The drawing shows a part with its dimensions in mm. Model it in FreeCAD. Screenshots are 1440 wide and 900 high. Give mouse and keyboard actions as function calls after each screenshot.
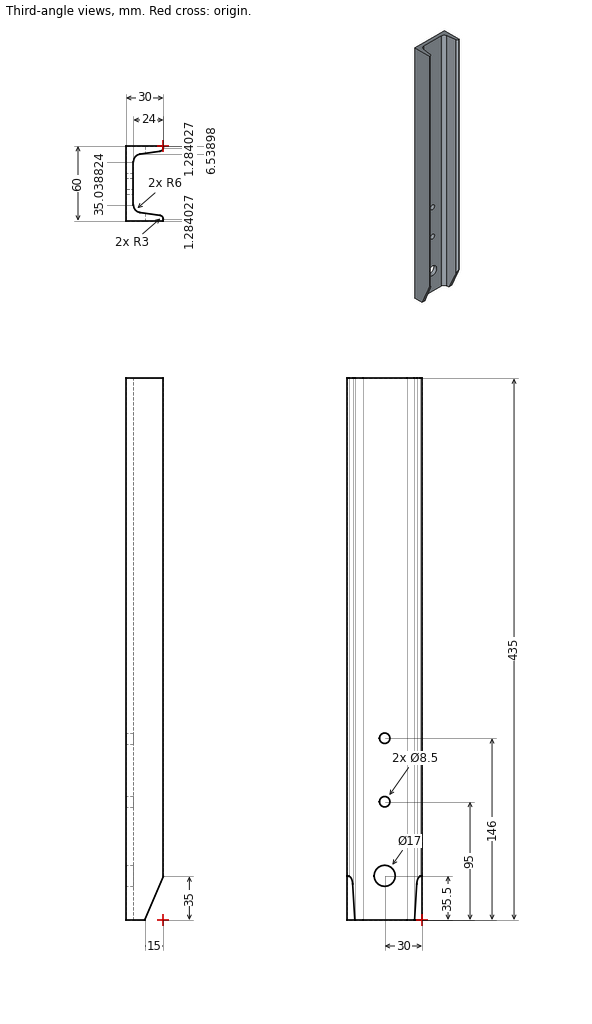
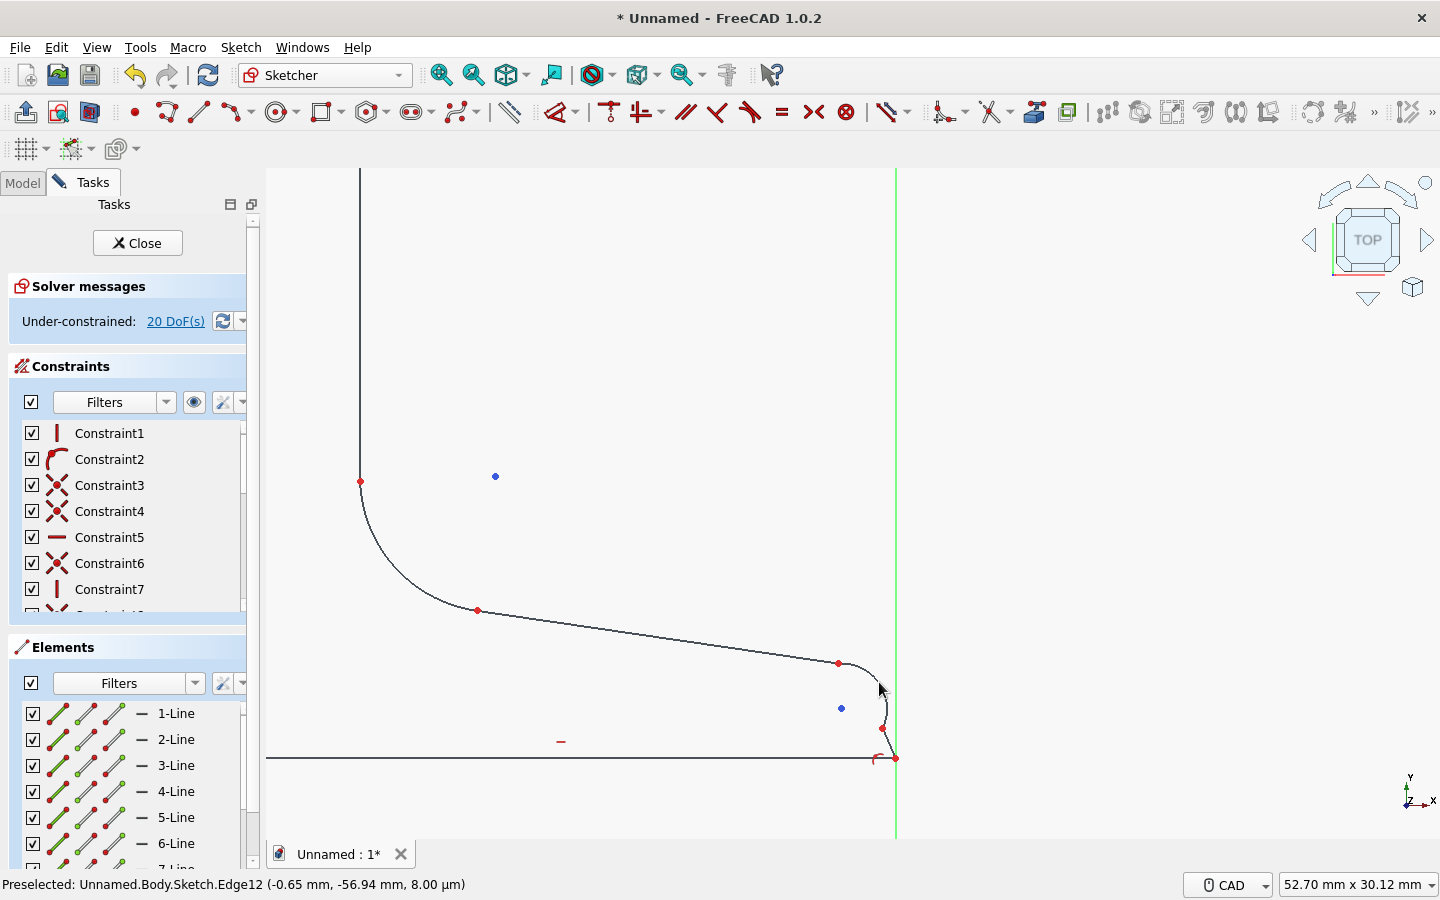
scroll(881, 683, down, 6)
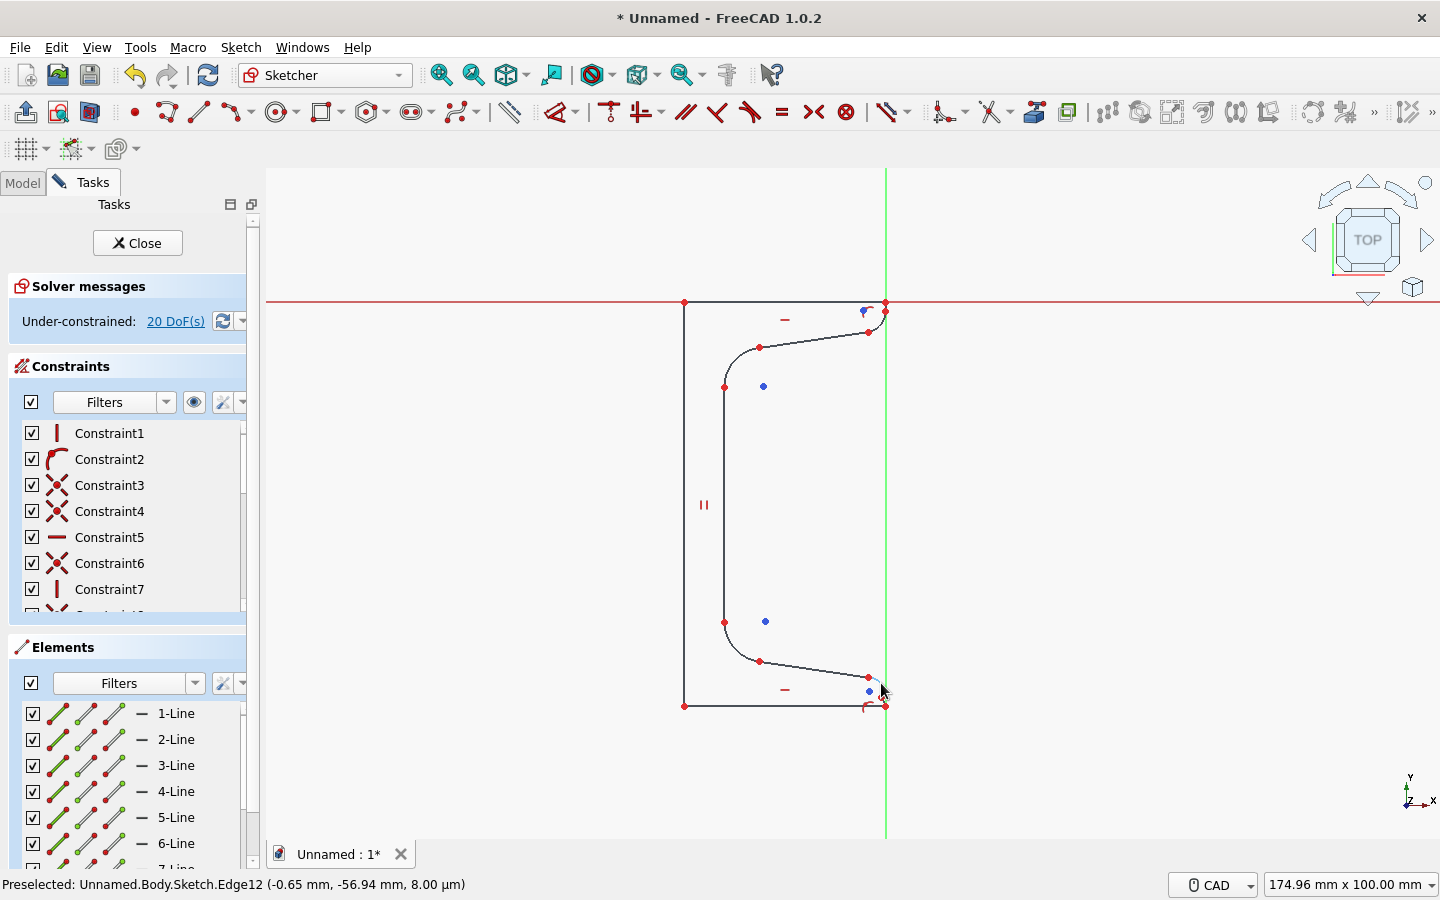
click(836, 673)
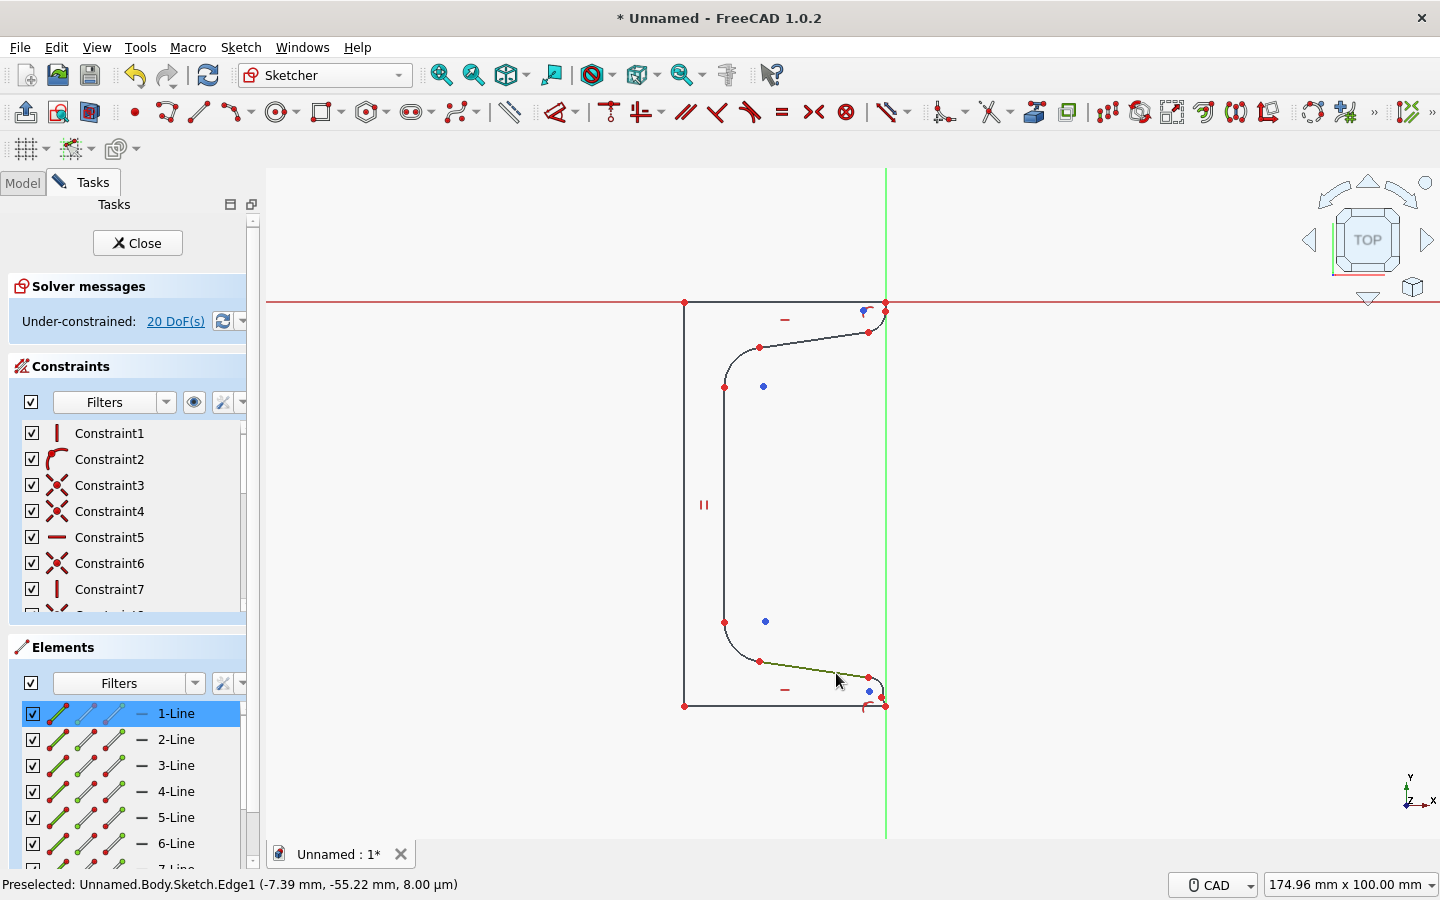
click(729, 639)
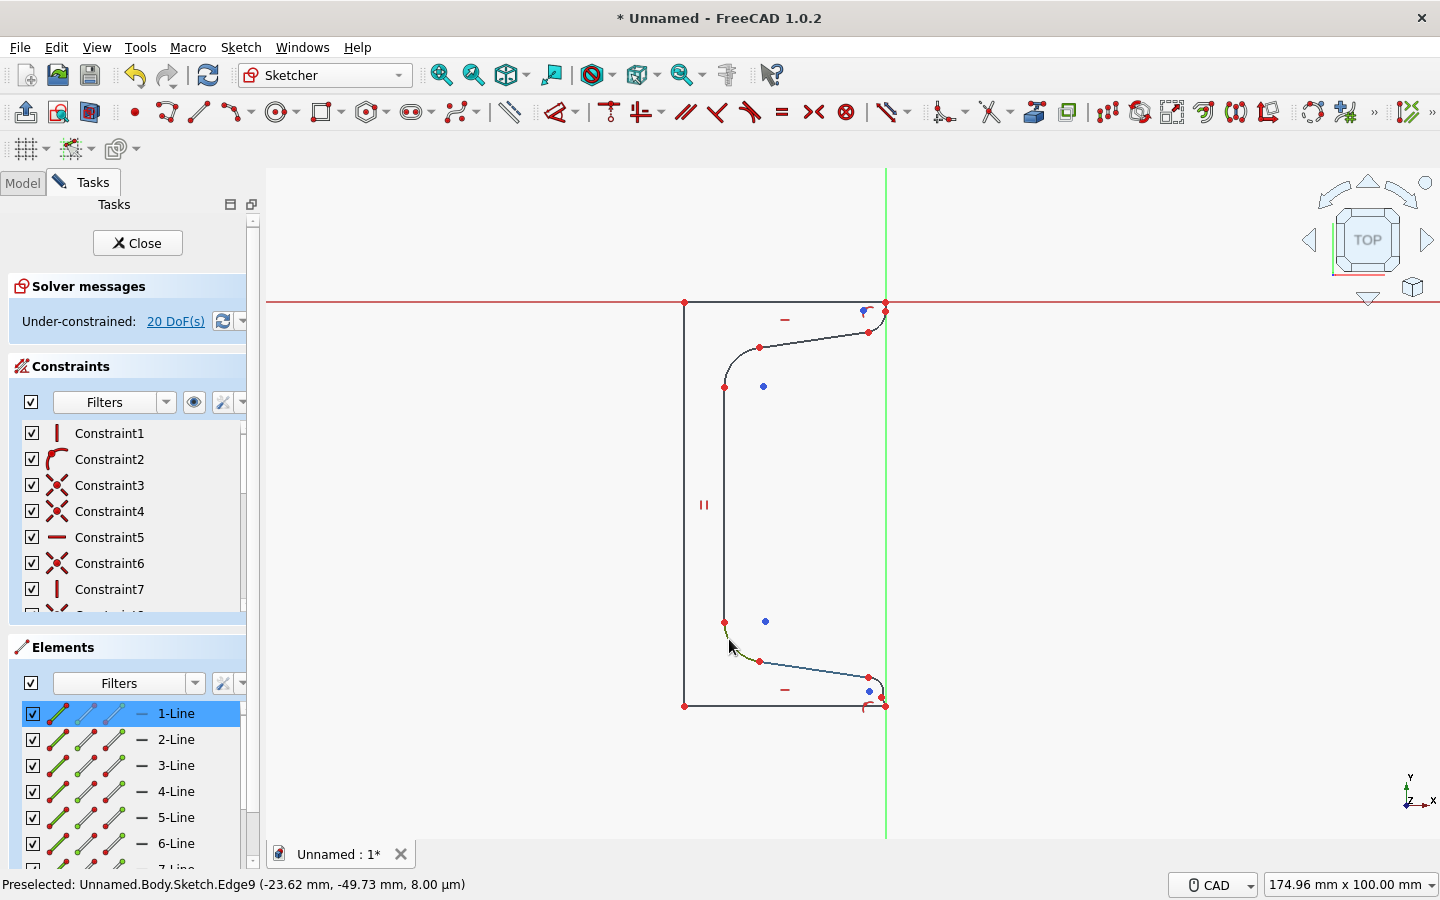
click(750, 112)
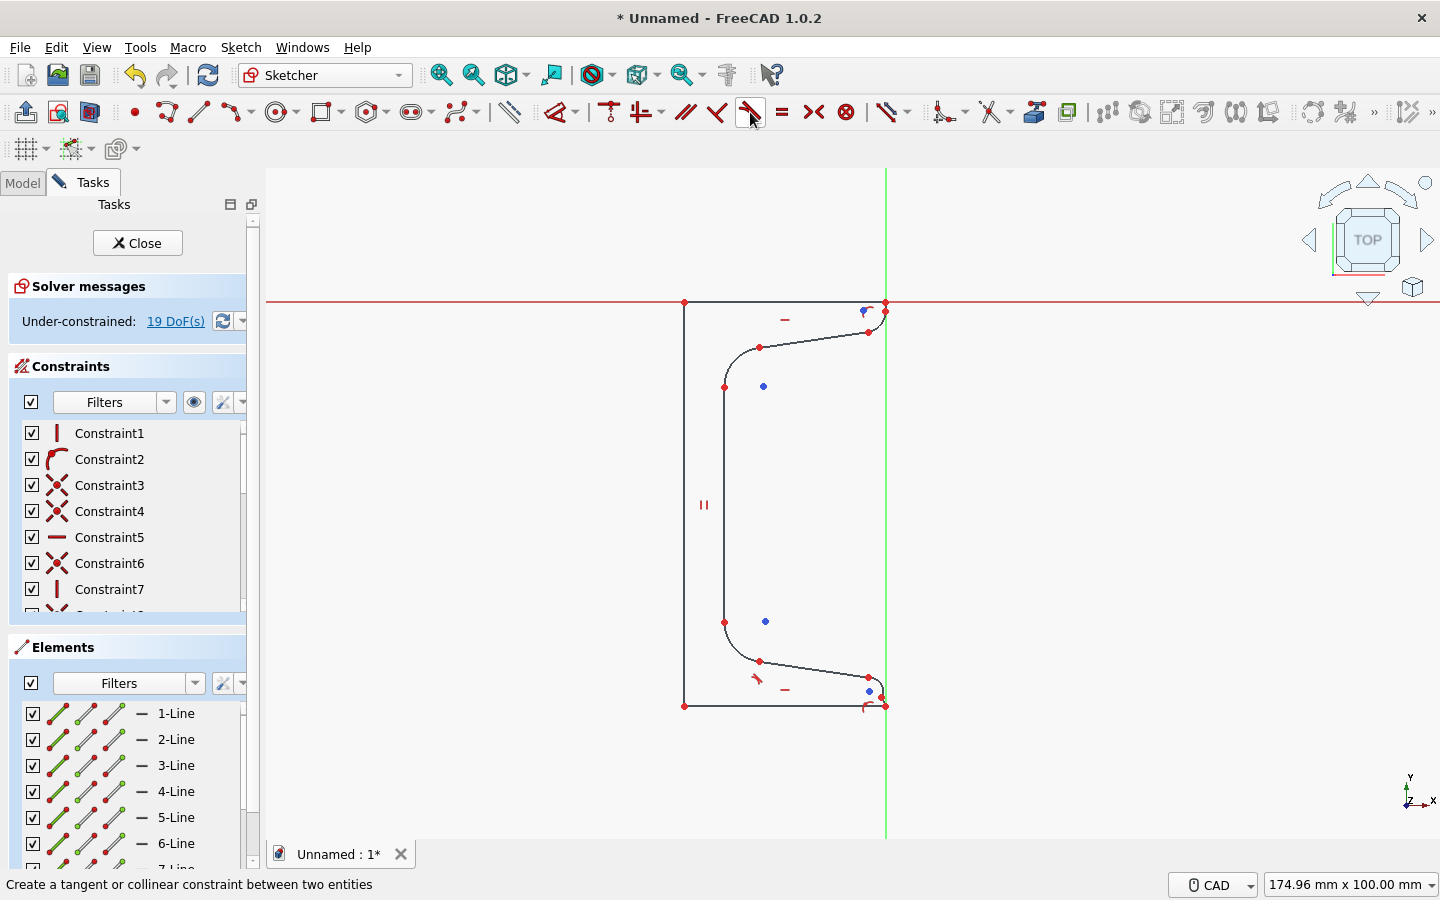
click(836, 673)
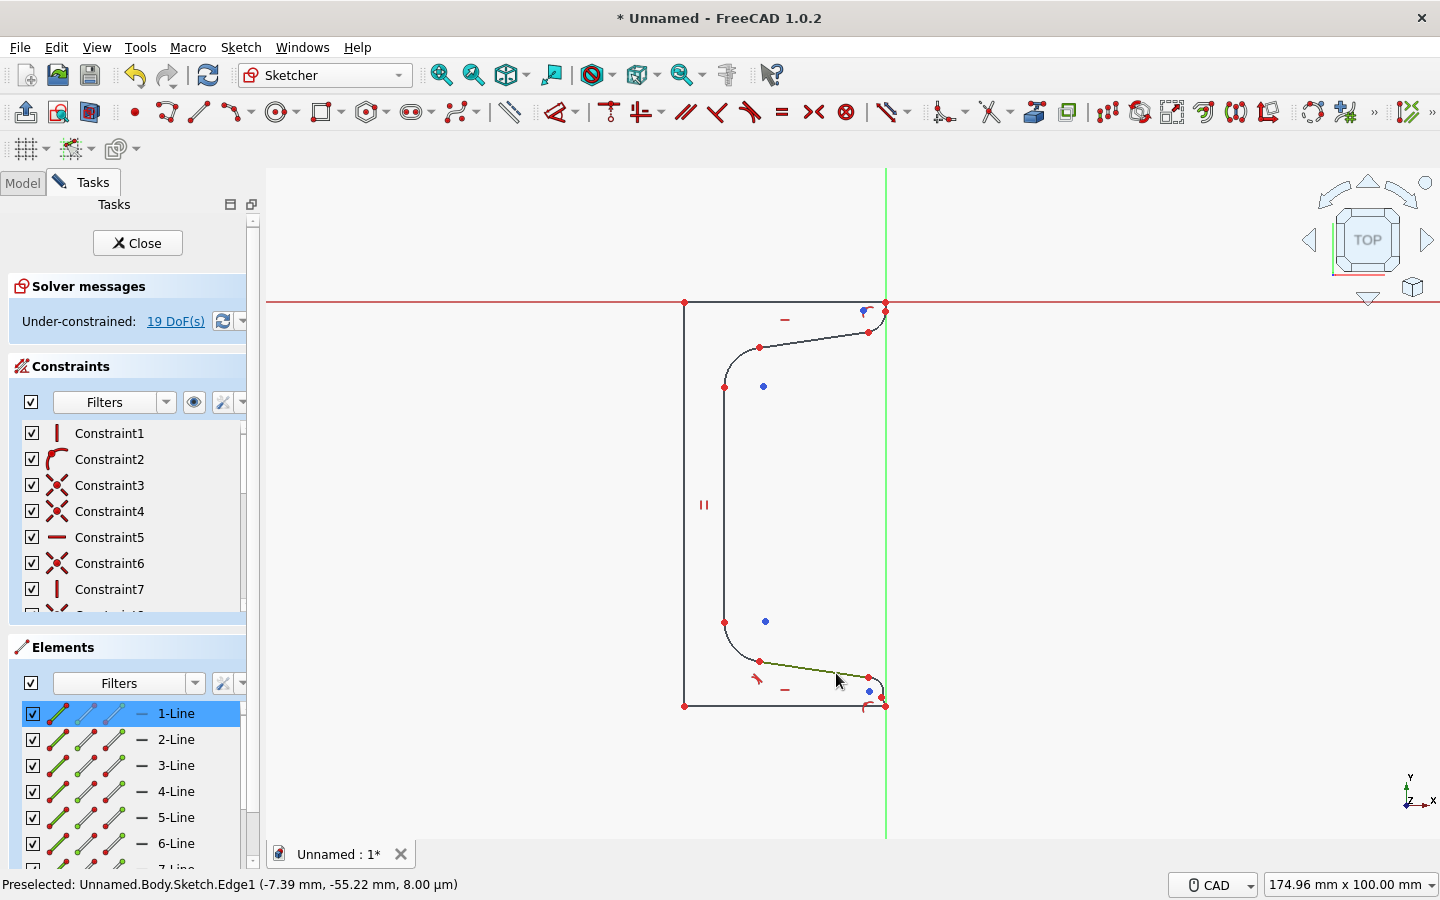
scroll(877, 680, up, 3)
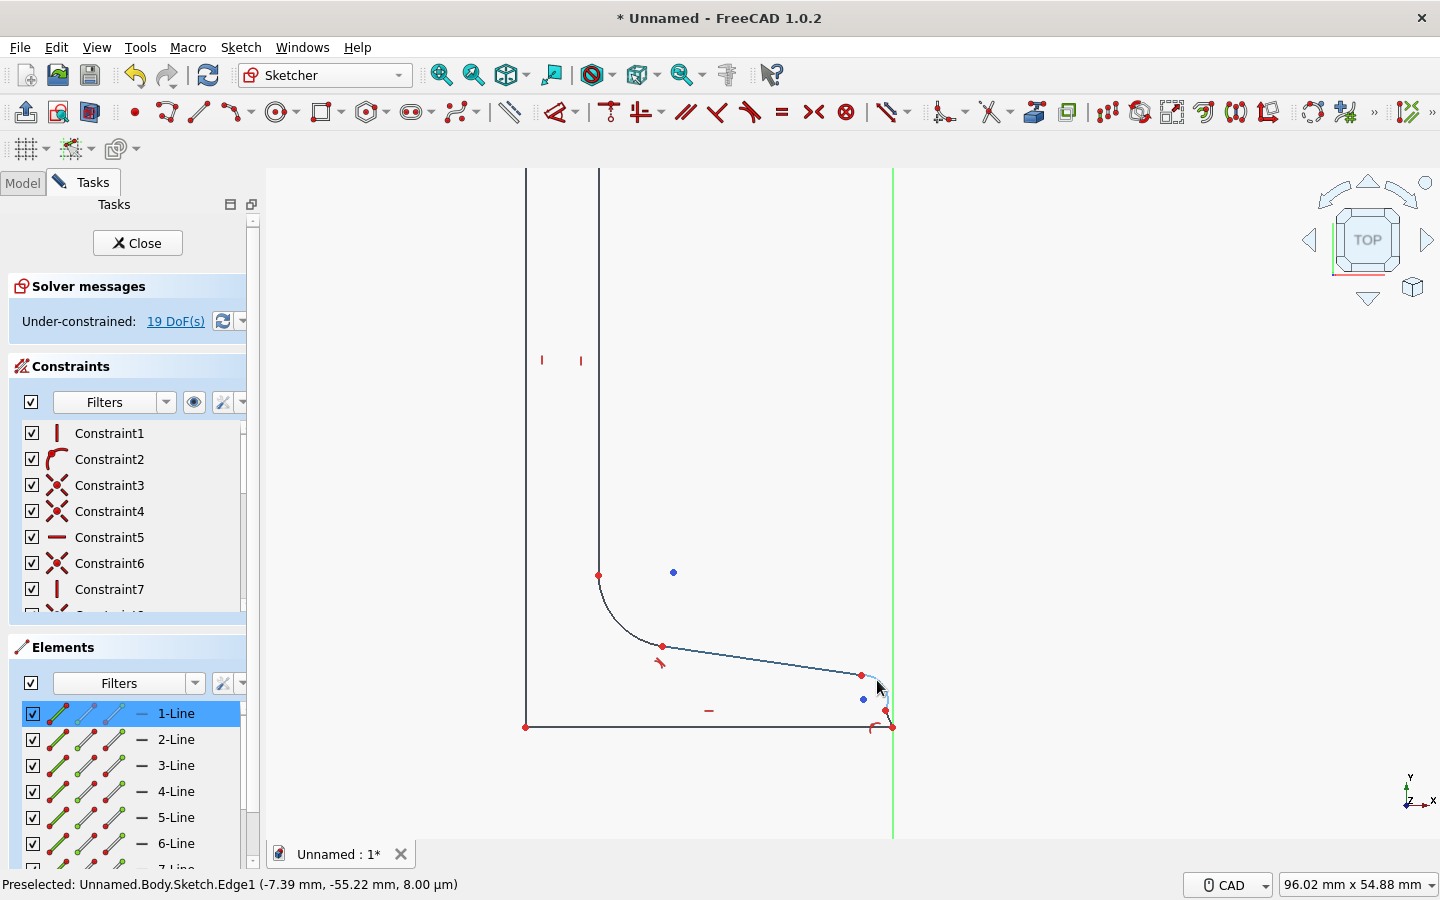
click(876, 679)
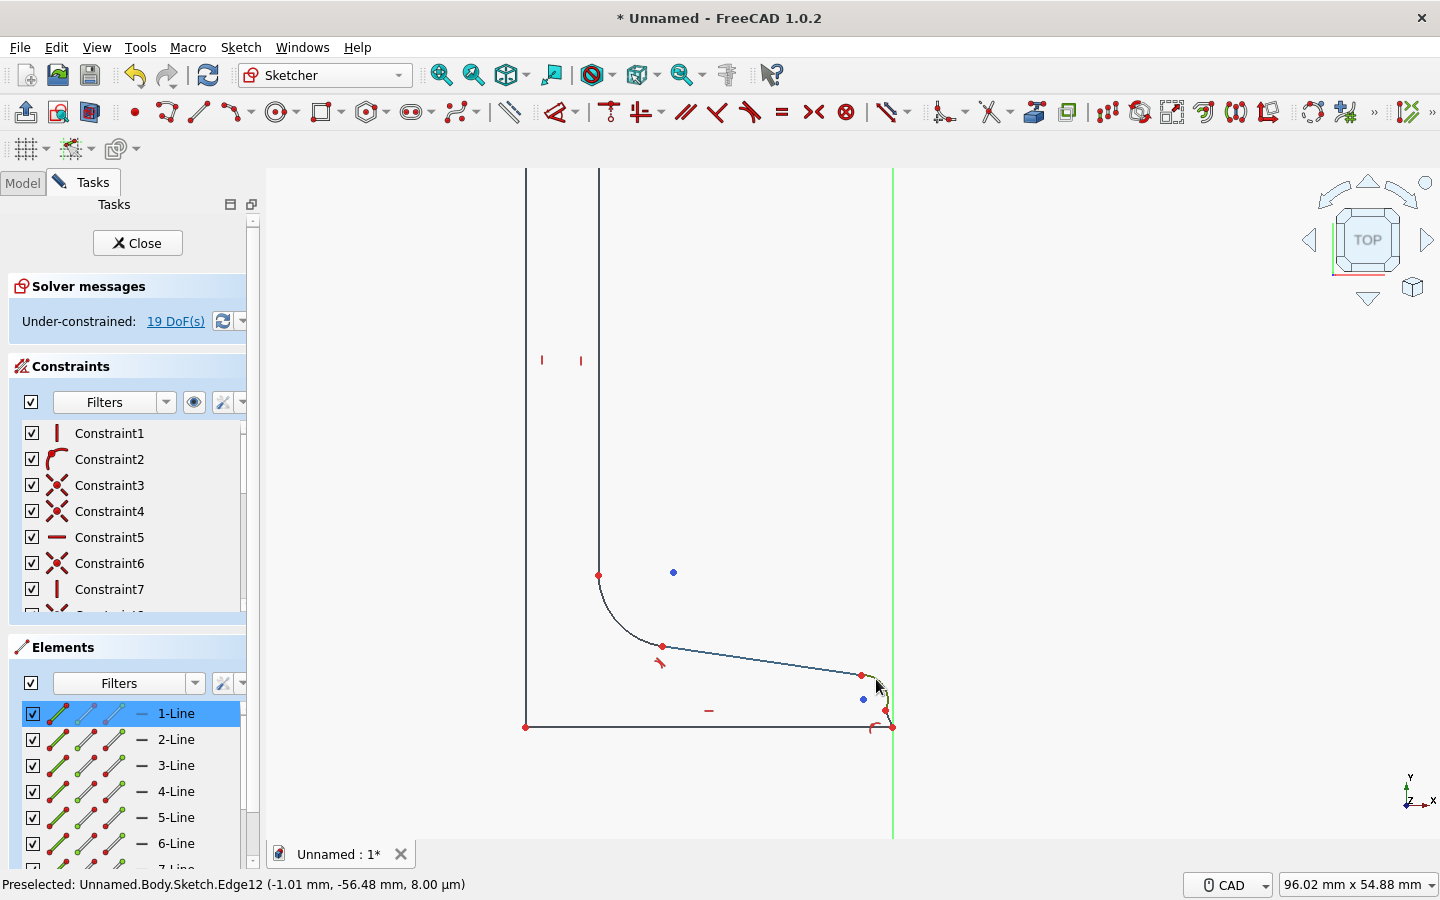
key(t)